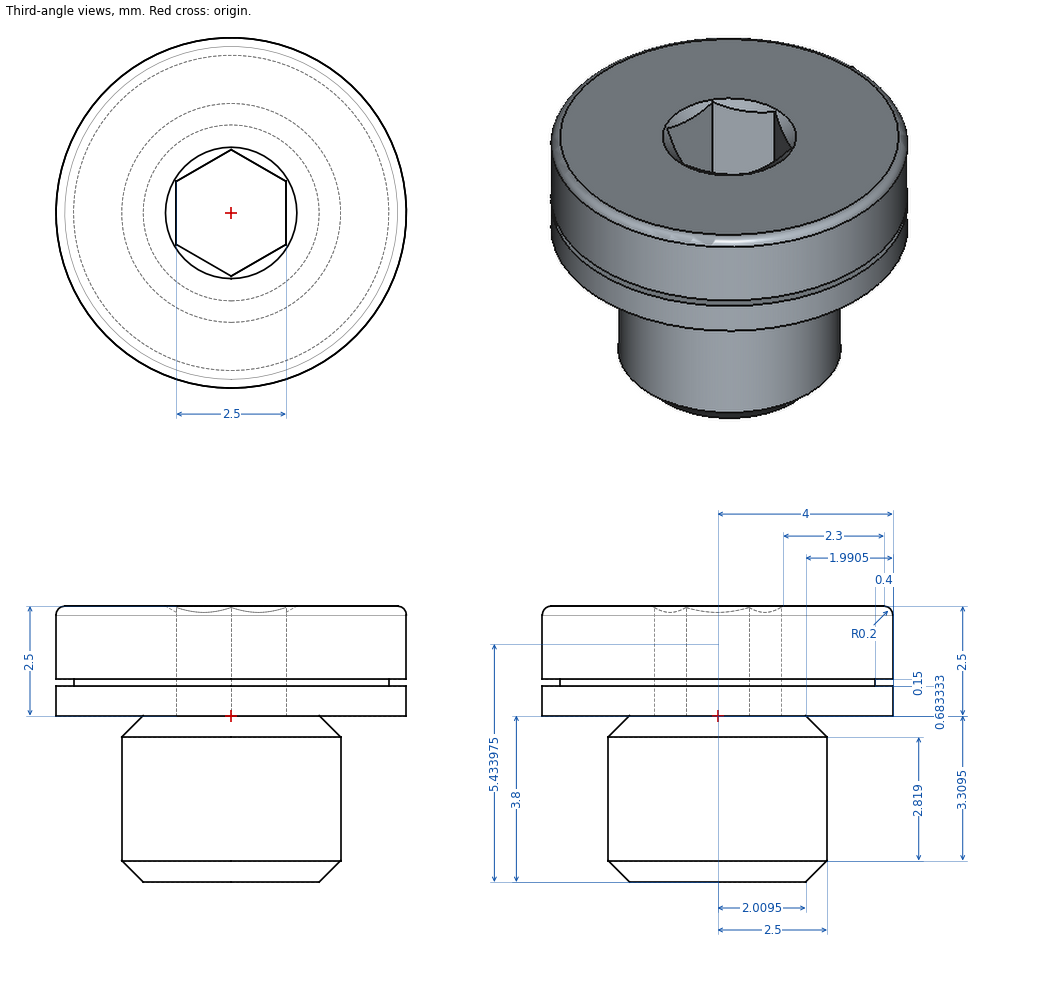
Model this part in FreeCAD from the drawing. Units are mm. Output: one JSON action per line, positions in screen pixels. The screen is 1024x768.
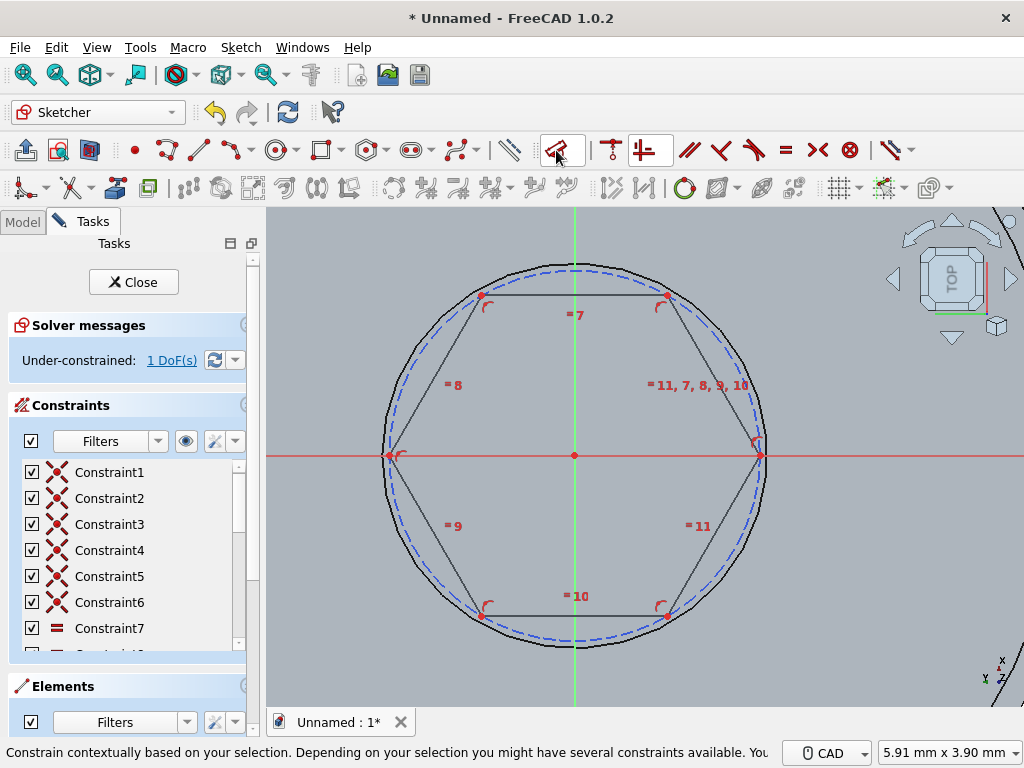
{"action": "left_click", "coordinate": [482, 616]}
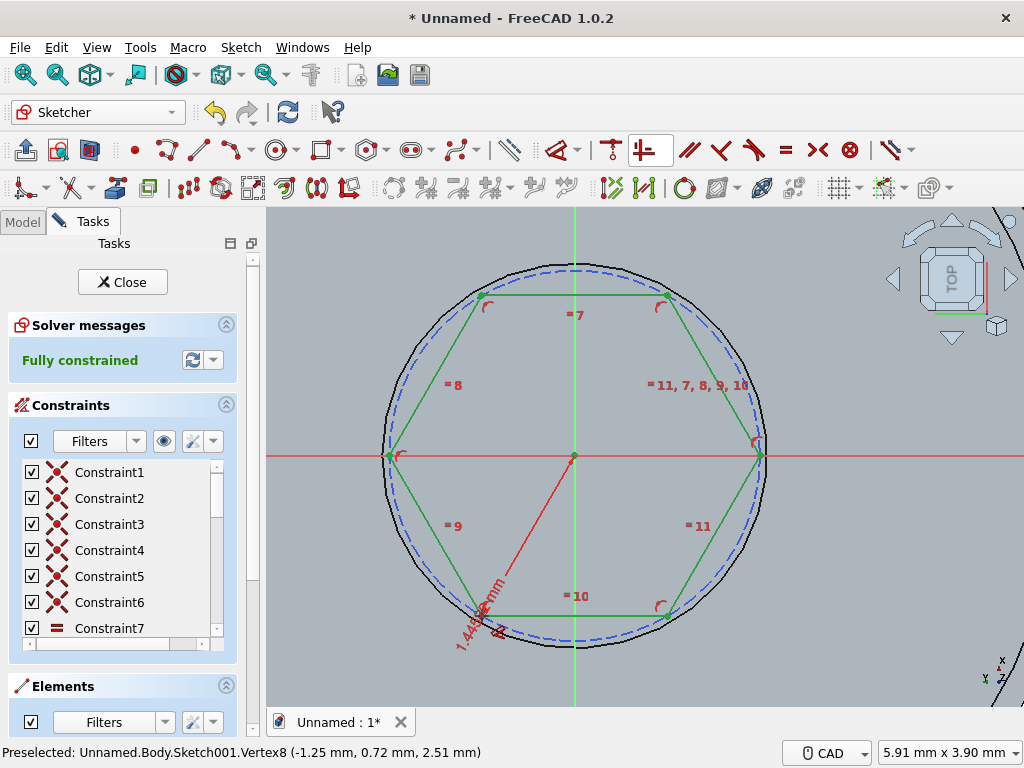
{"action": "left_click", "coordinate": [667, 295]}
{"action": "left_click", "coordinate": [701, 382]}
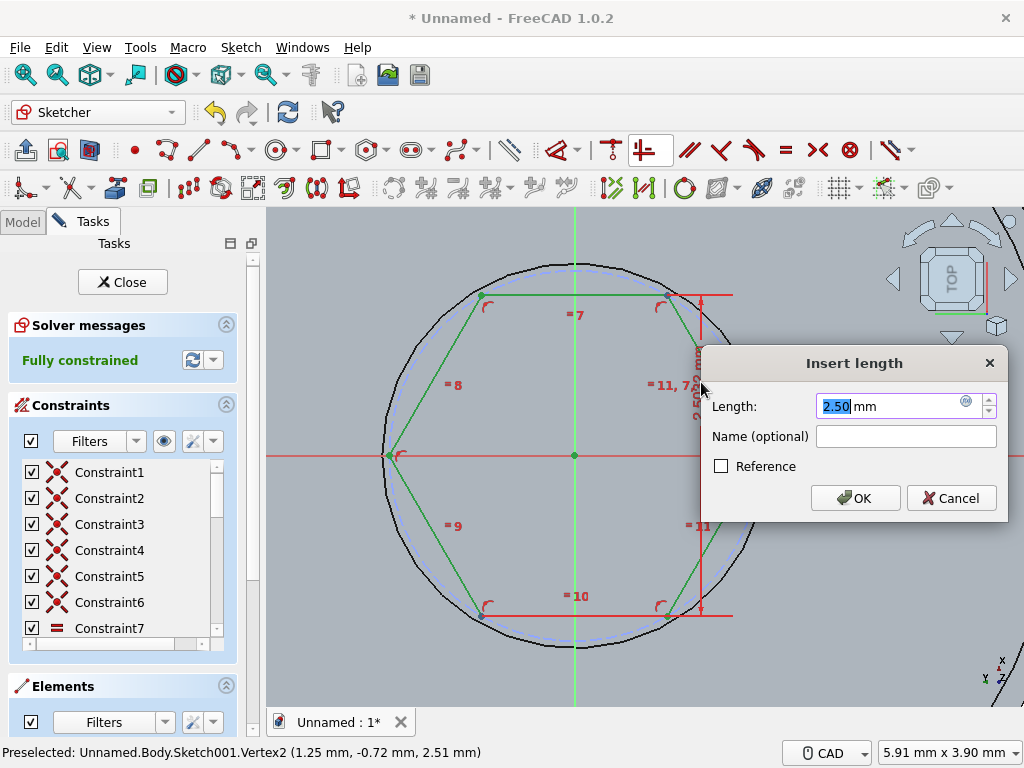
{"action": "type", "text": "2.5"}
{"action": "key", "text": "Return"}
{"action": "key", "text": "Escape"}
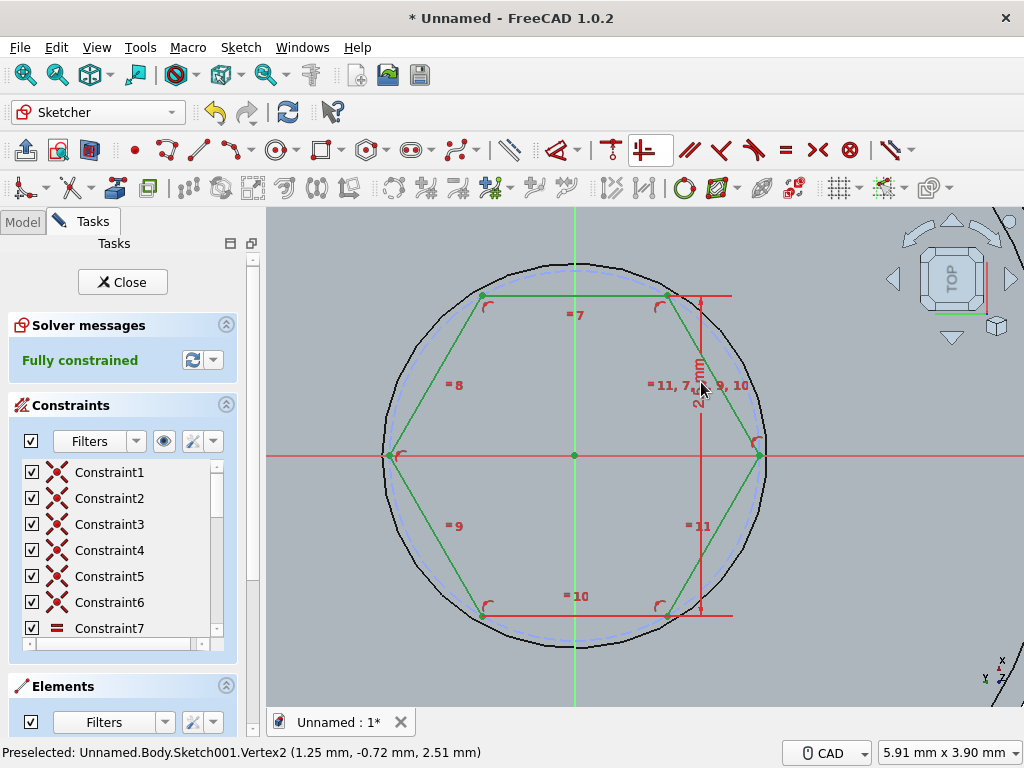
{"action": "left_click", "coordinate": [123, 282]}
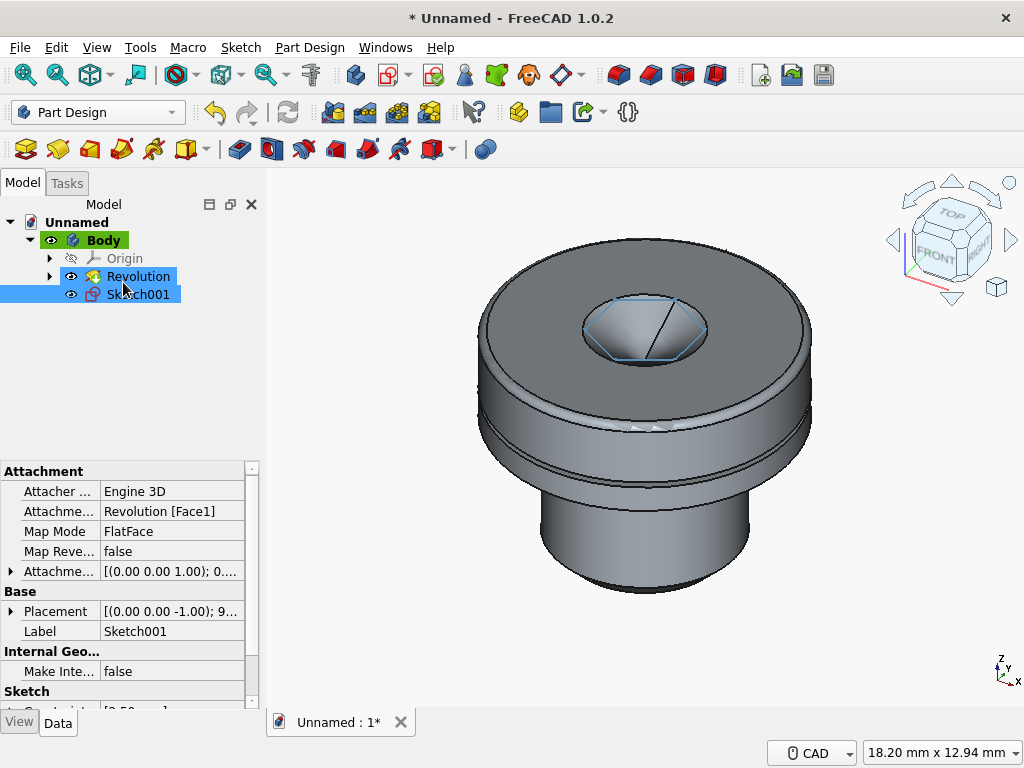
{"action": "left_click", "coordinate": [240, 150]}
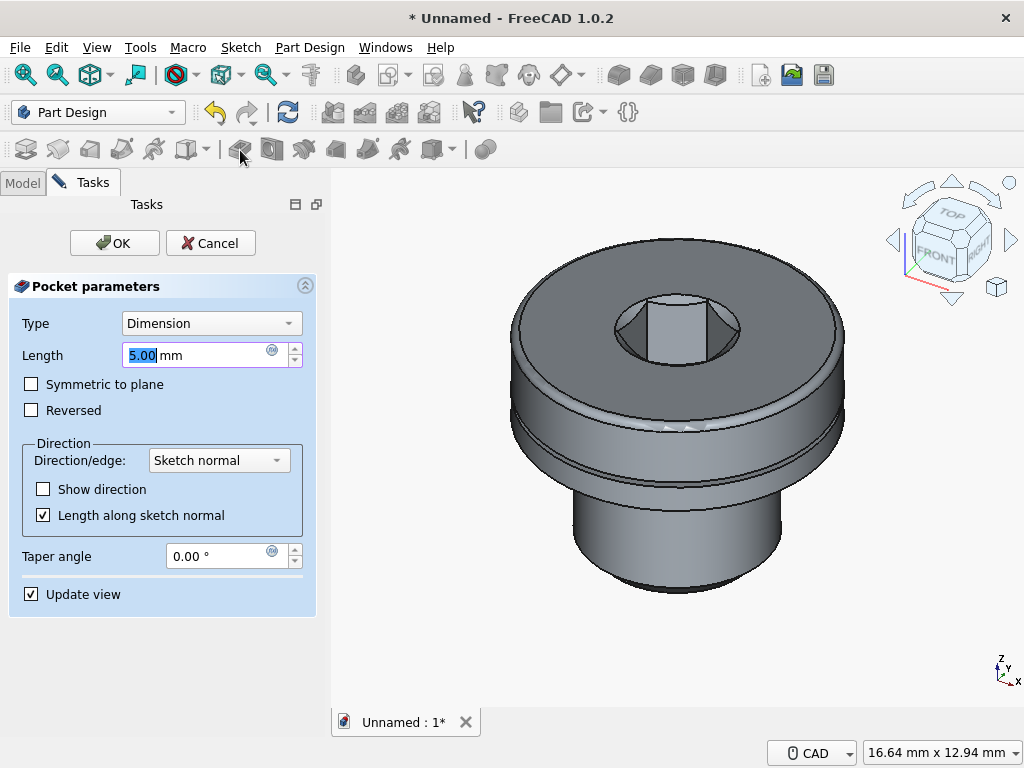
{"action": "type", "text": "2.5"}
{"action": "key", "text": "Tab"}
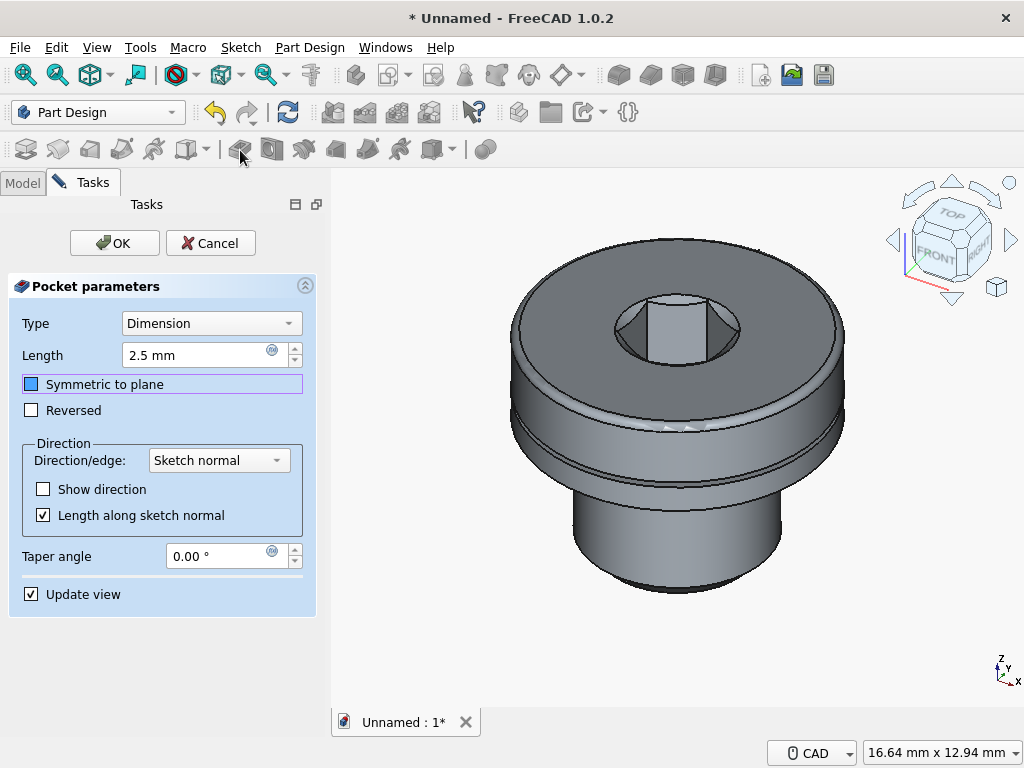
{"action": "left_click", "coordinate": [115, 243]}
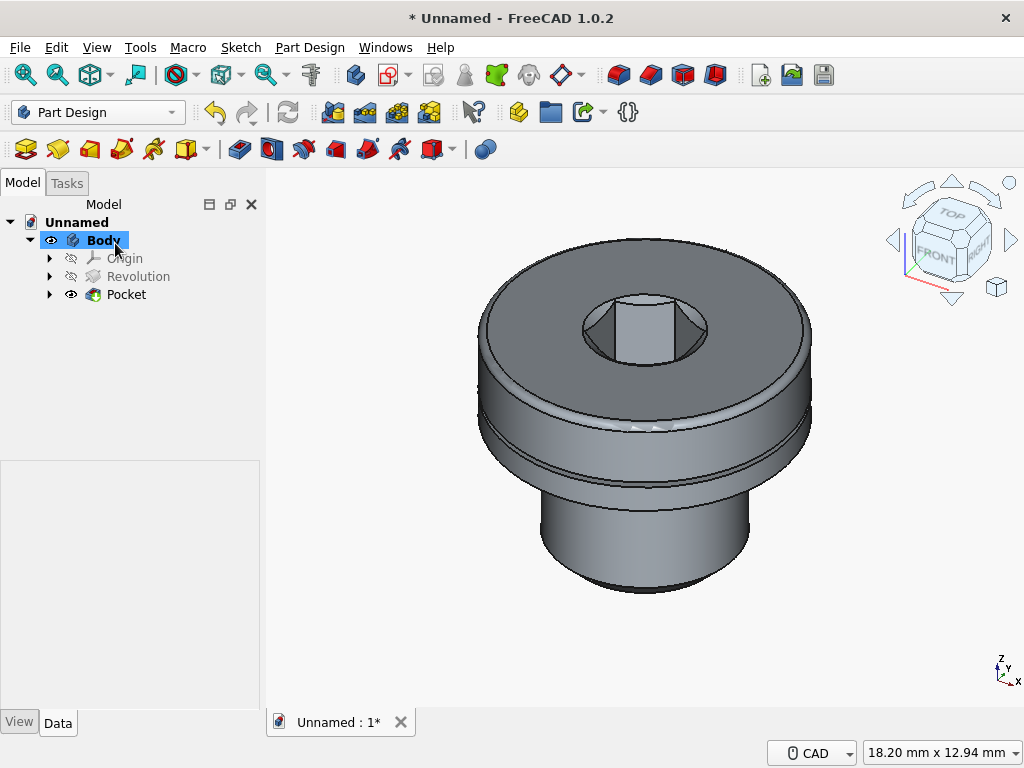
{"action": "key", "text": "0"}